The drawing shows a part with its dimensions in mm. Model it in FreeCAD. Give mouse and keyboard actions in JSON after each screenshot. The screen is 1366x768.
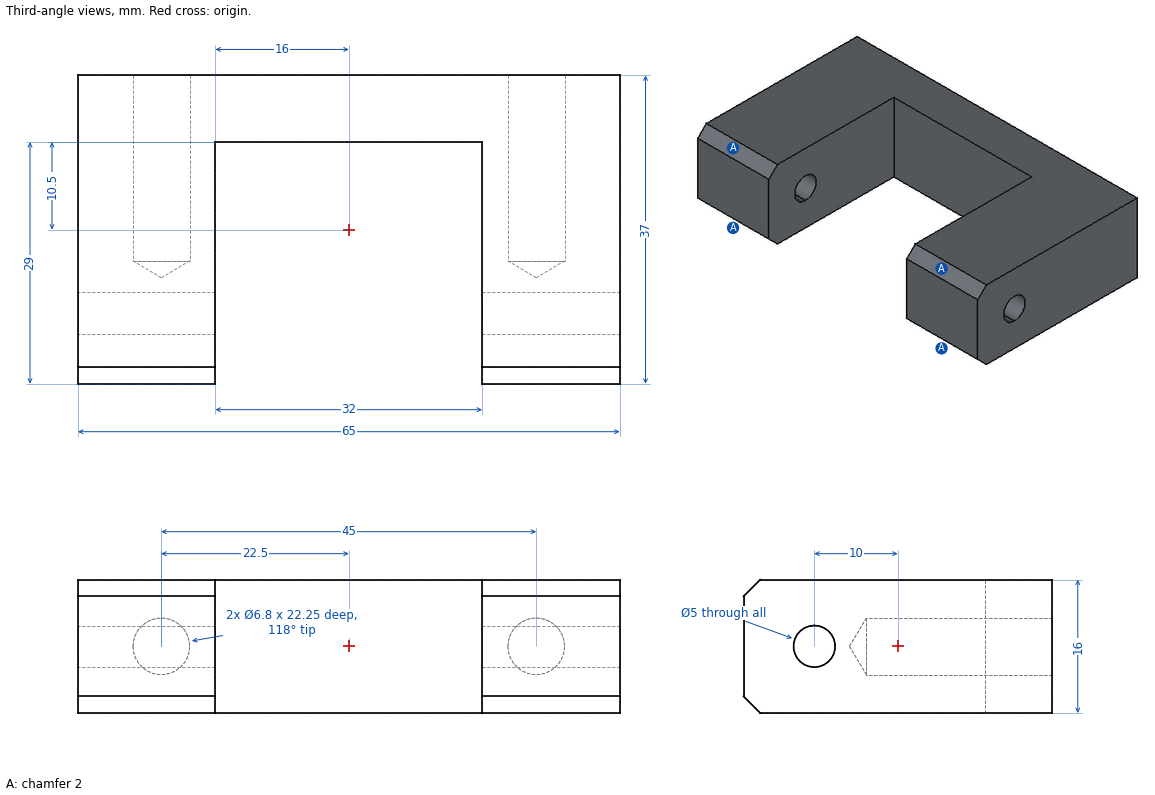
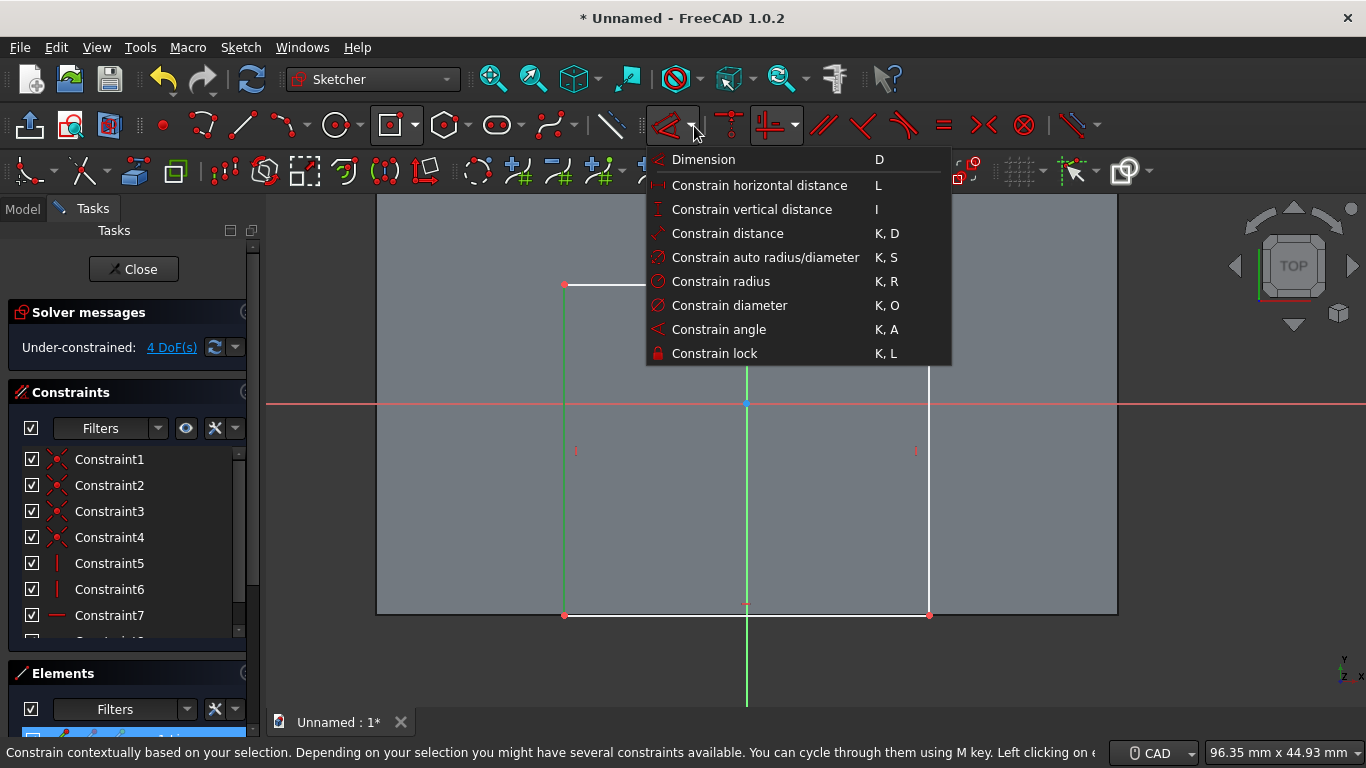
{"action": "left_click", "coordinate": [799, 209]}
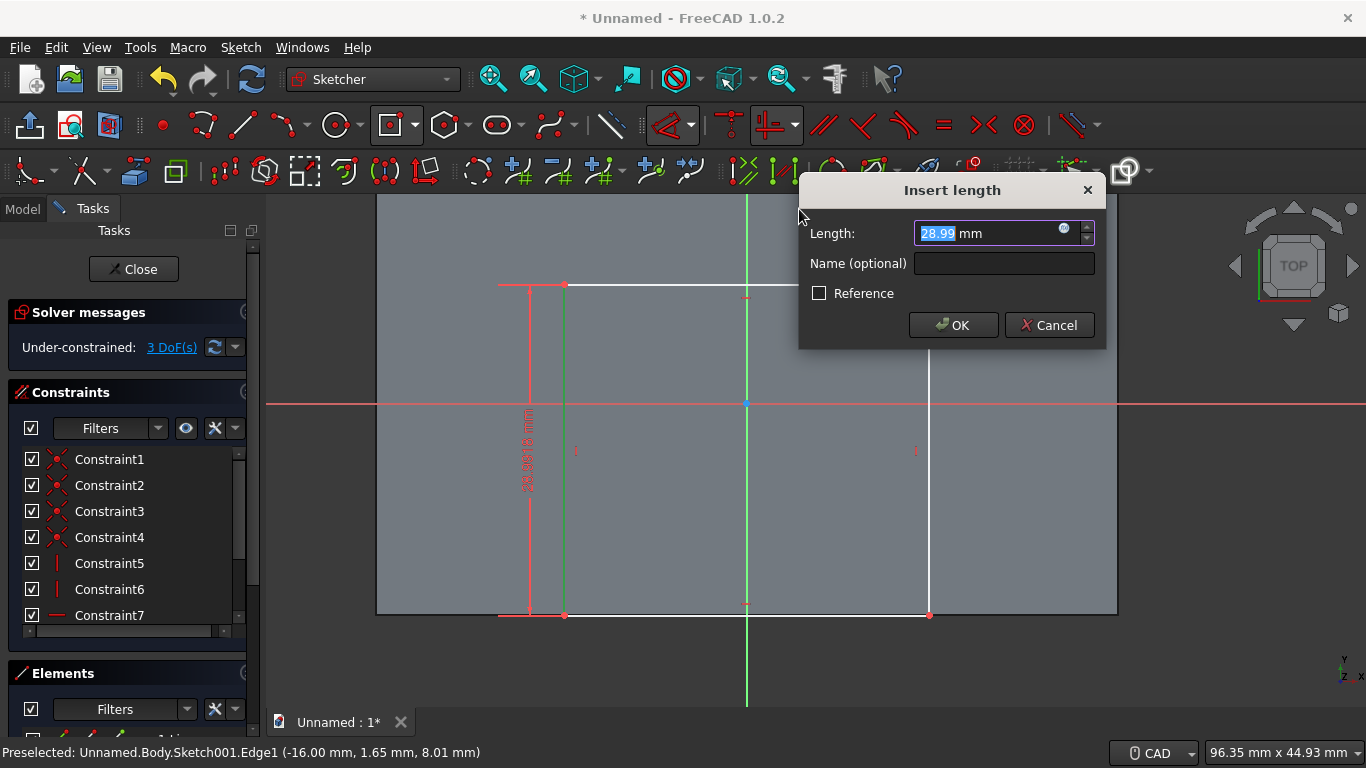
{"action": "type", "text": "29"}
{"action": "key", "text": "Return"}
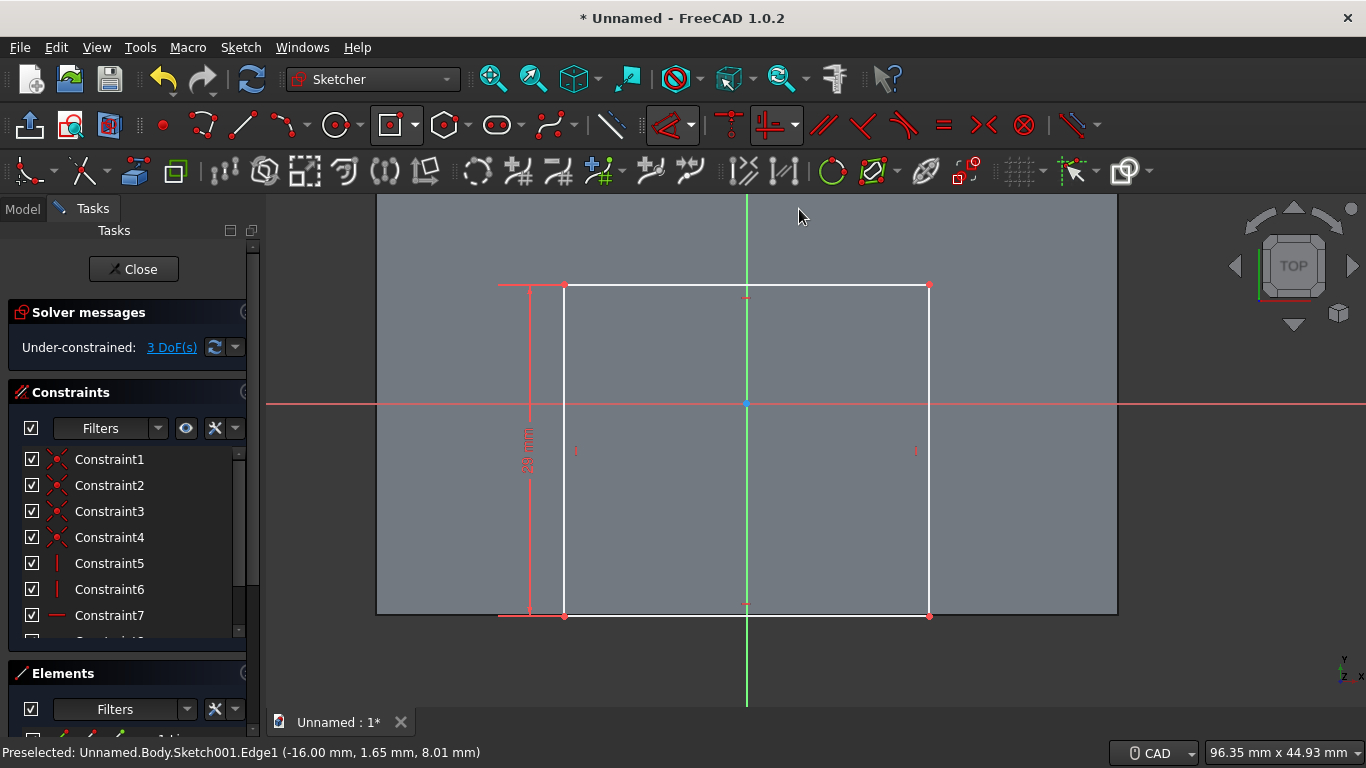
{"action": "left_click", "coordinate": [674, 616]}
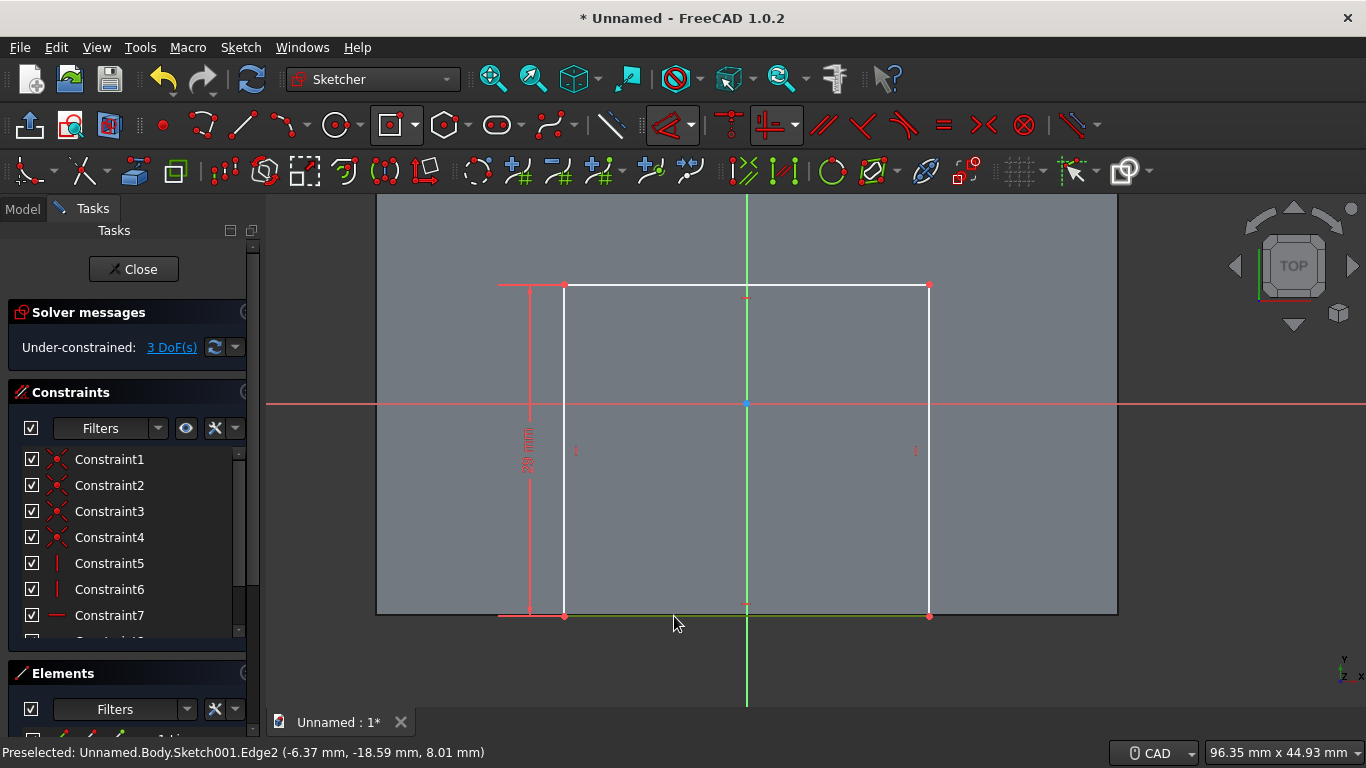
{"action": "key", "text": "l"}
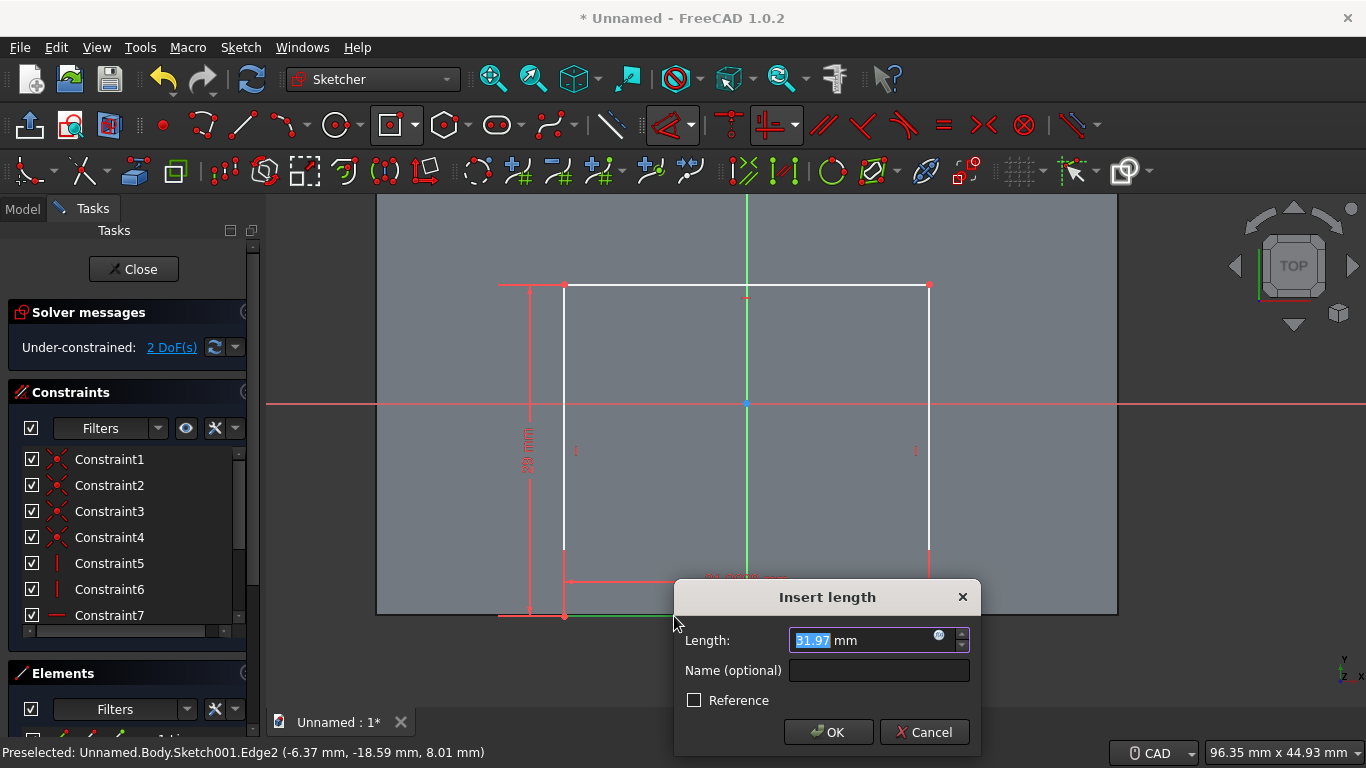
{"action": "type", "text": "32"}
{"action": "key", "text": "Return"}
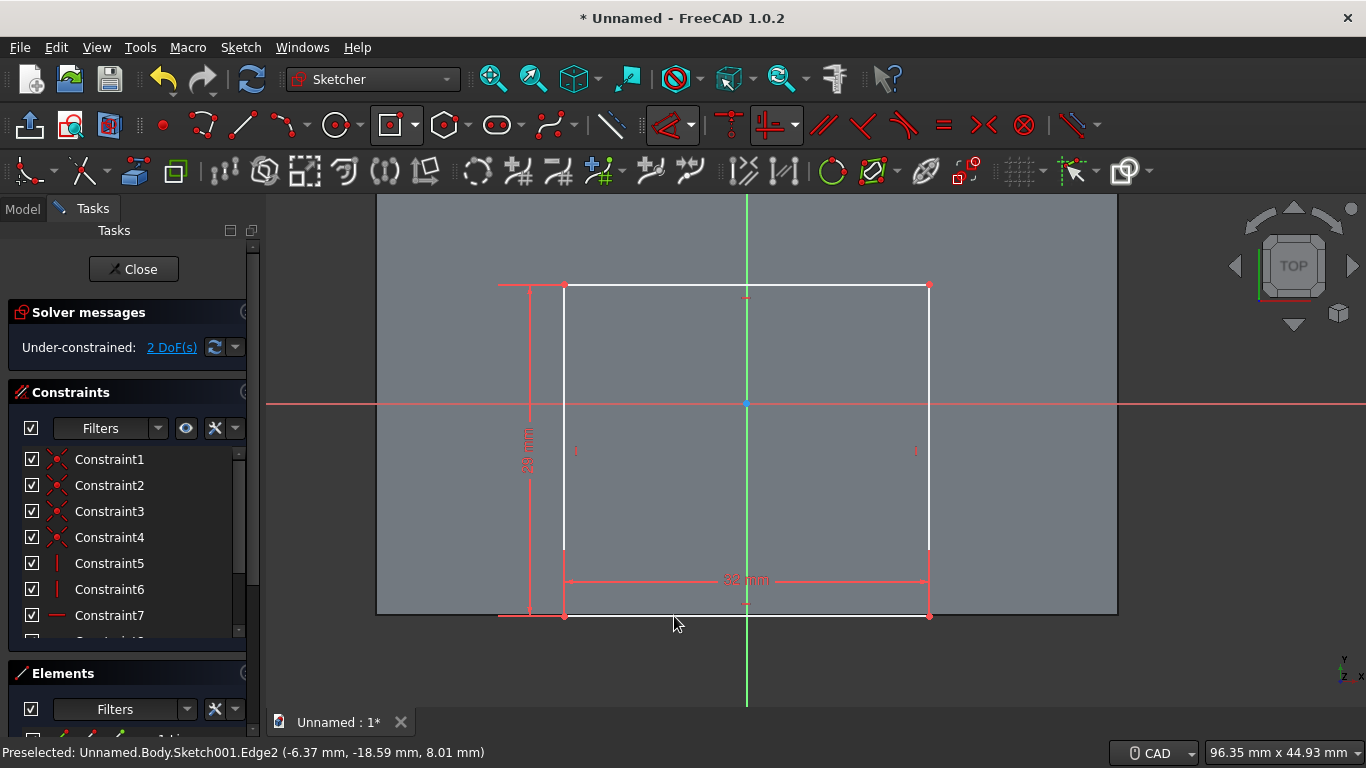
{"action": "left_click", "coordinate": [564, 285]}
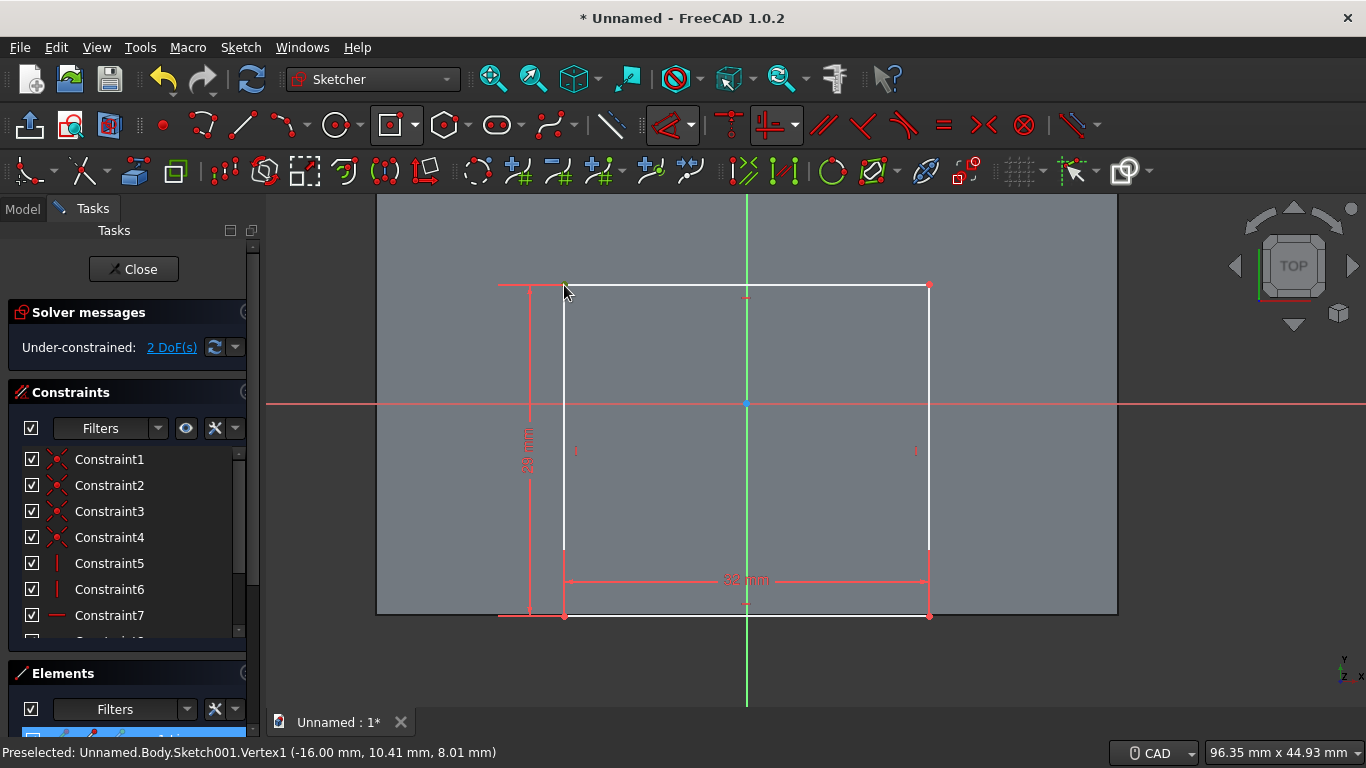
{"action": "key", "text": "l"}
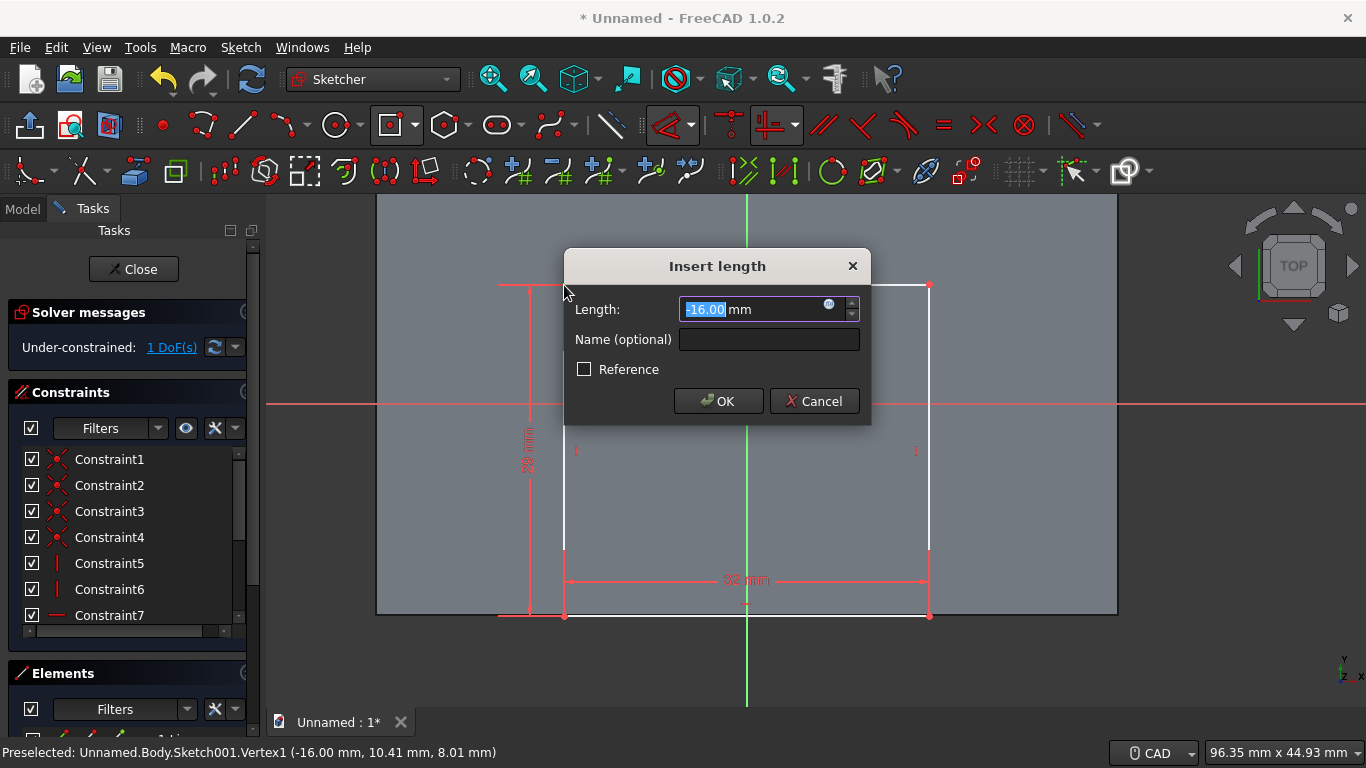
{"action": "type", "text": "-16"}
{"action": "key", "text": "Return"}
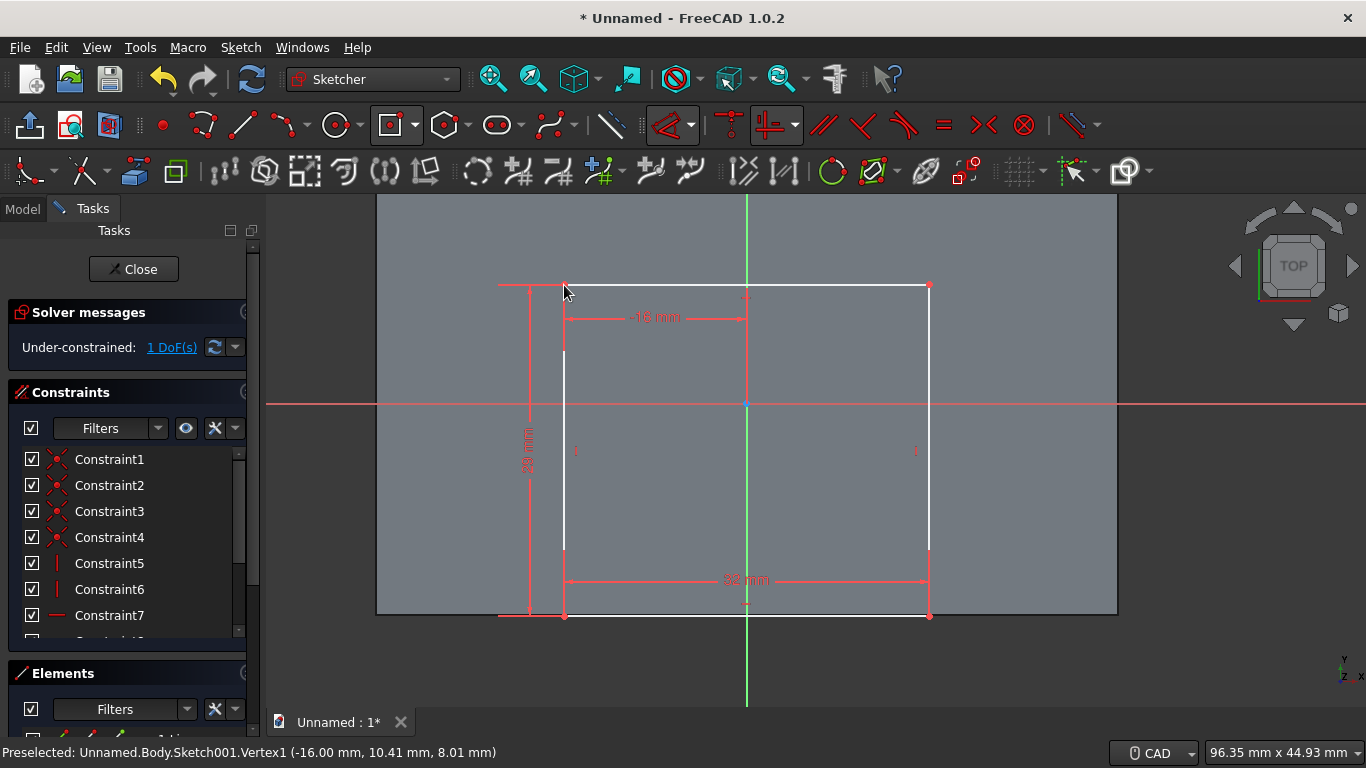
{"action": "left_click", "coordinate": [564, 285]}